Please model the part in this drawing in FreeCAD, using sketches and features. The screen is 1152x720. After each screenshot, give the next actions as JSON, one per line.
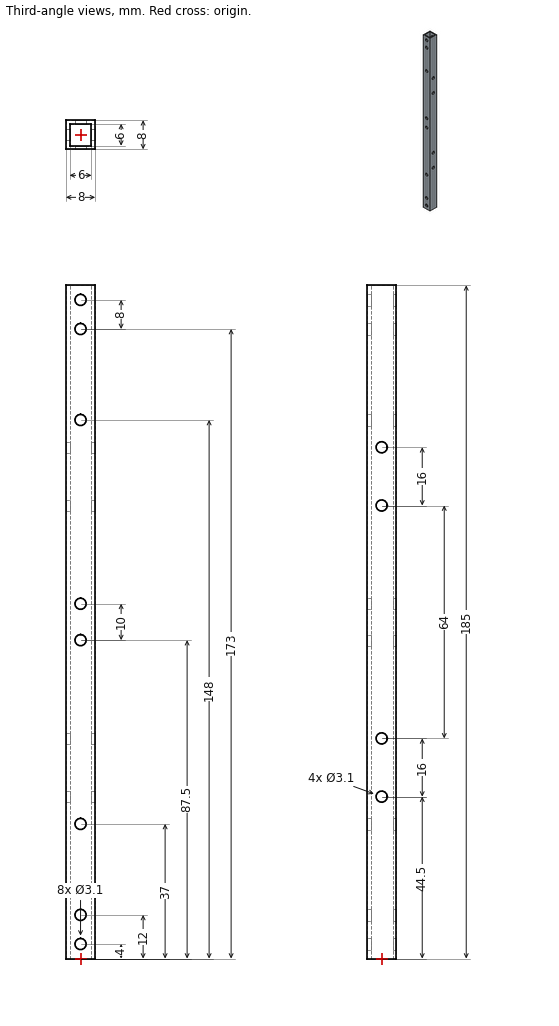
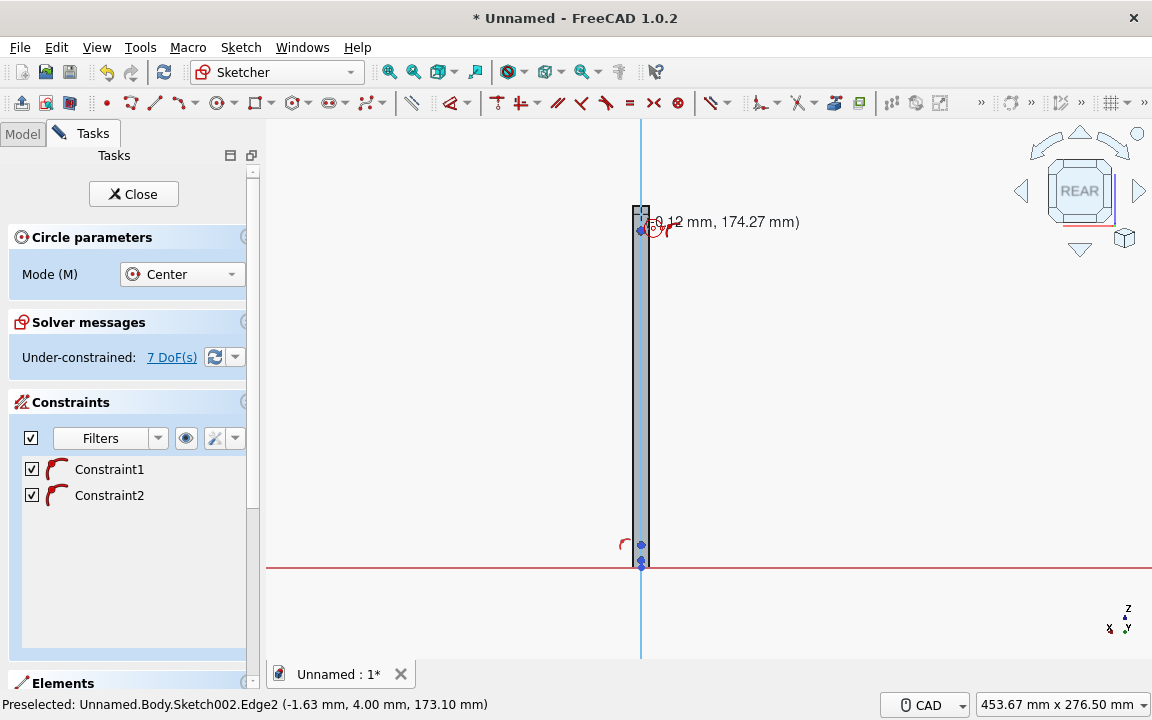
{"action": "scroll", "coordinate": [641, 214], "scroll_direction": "up", "scroll_amount": 2}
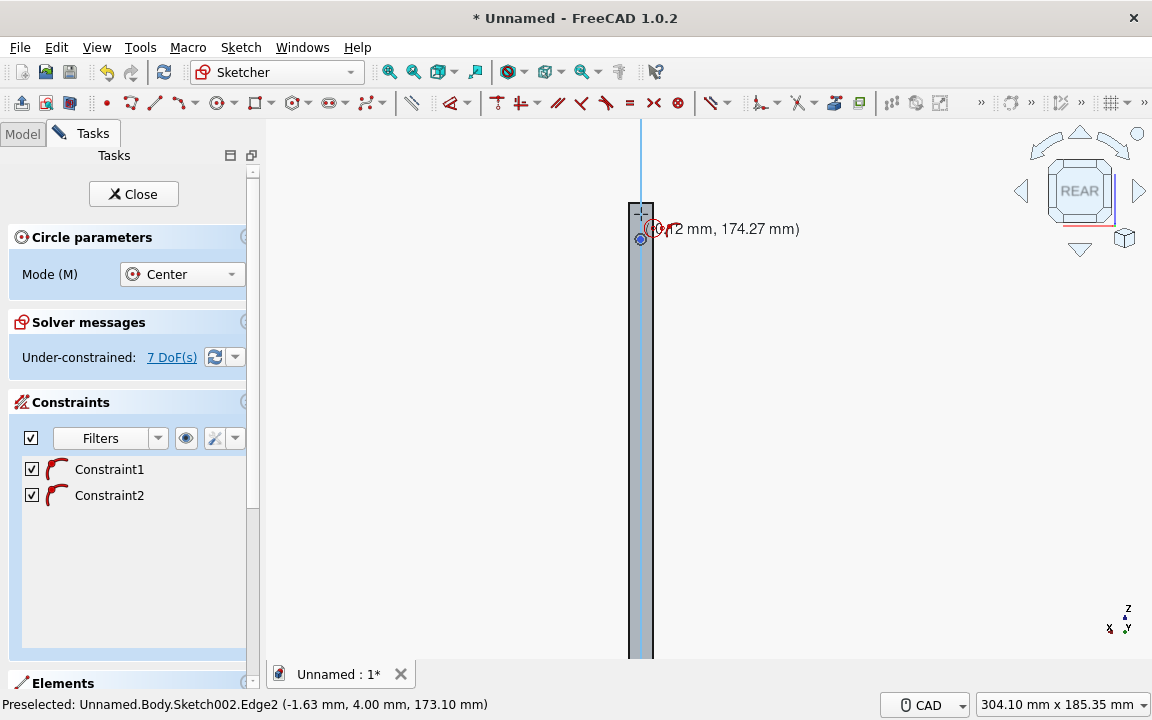
{"action": "left_click", "coordinate": [641, 214]}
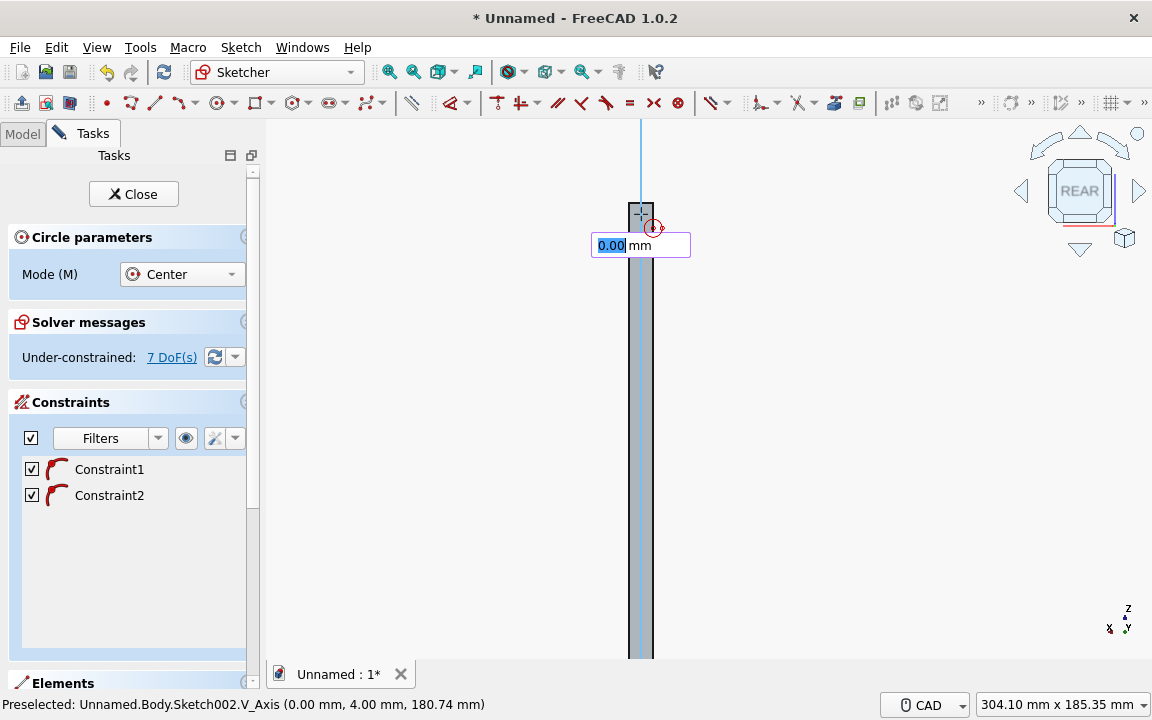
{"action": "scroll", "coordinate": [645, 213], "scroll_direction": "up", "scroll_amount": 7}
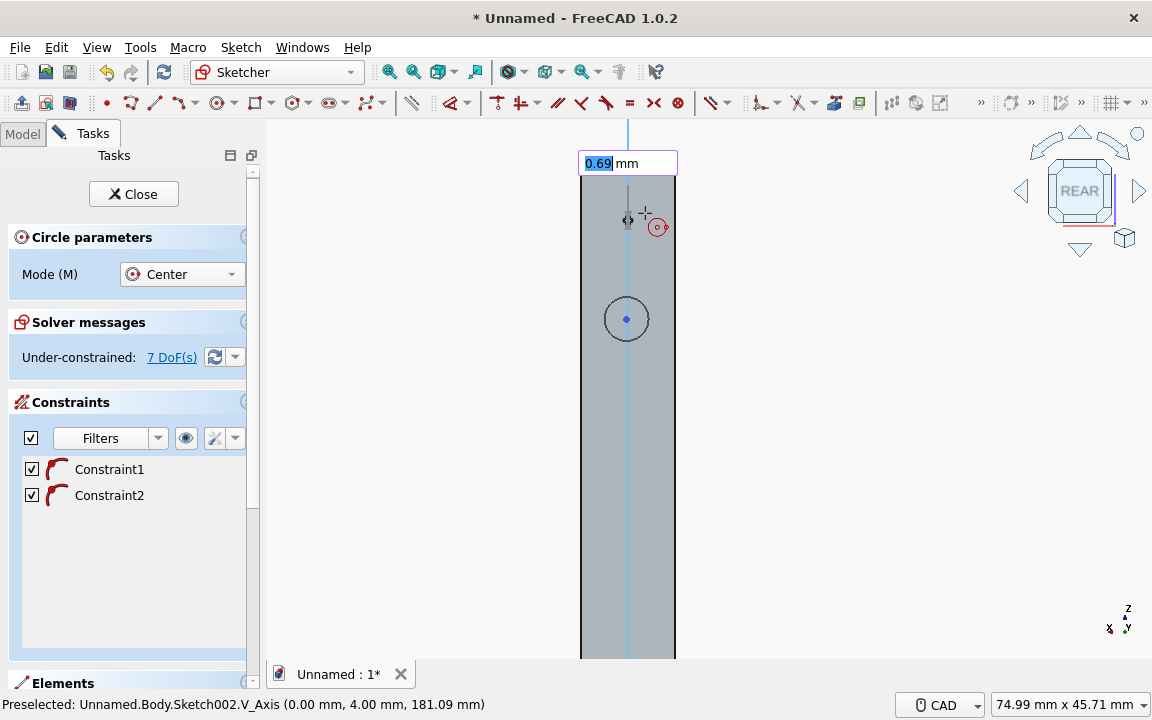
{"action": "left_click", "coordinate": [645, 211]}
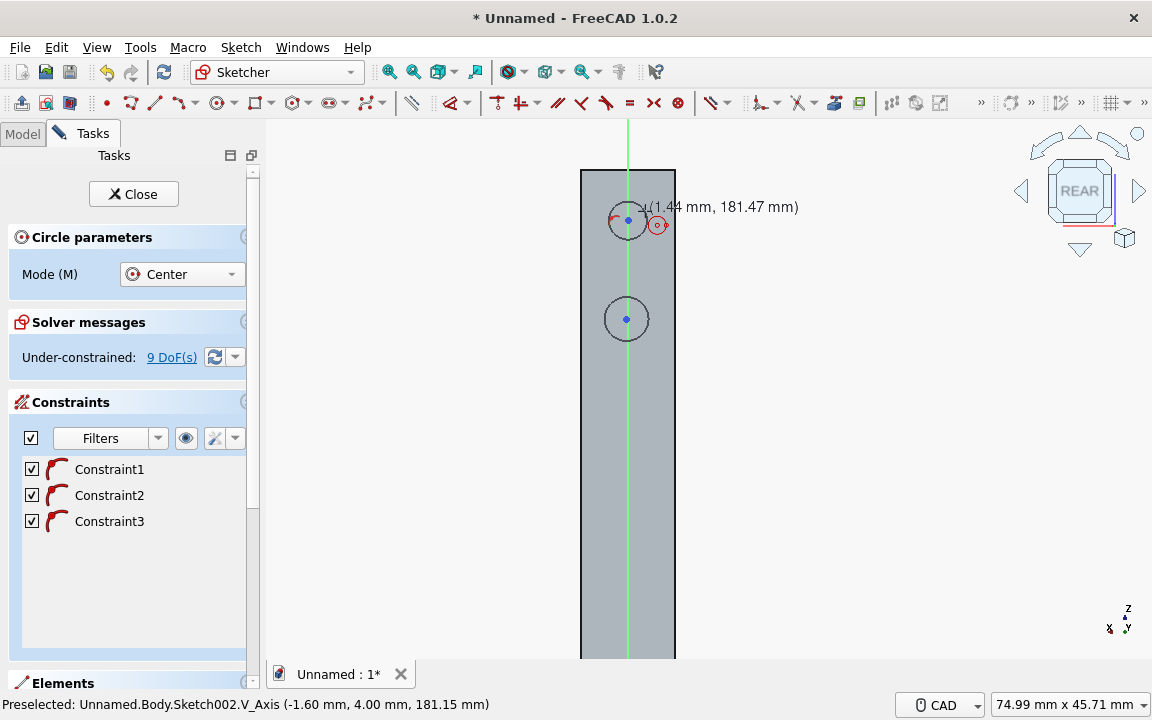
{"action": "scroll", "coordinate": [643, 213], "scroll_direction": "down", "scroll_amount": 9}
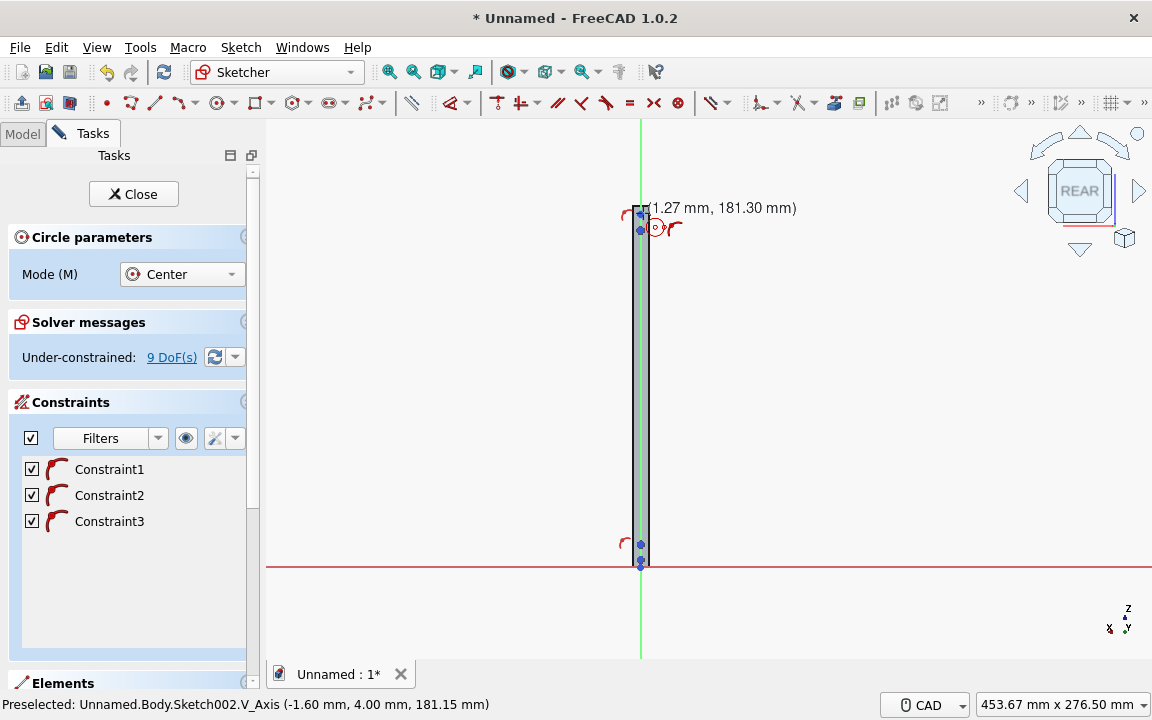
{"action": "scroll", "coordinate": [641, 396], "scroll_direction": "up", "scroll_amount": 11}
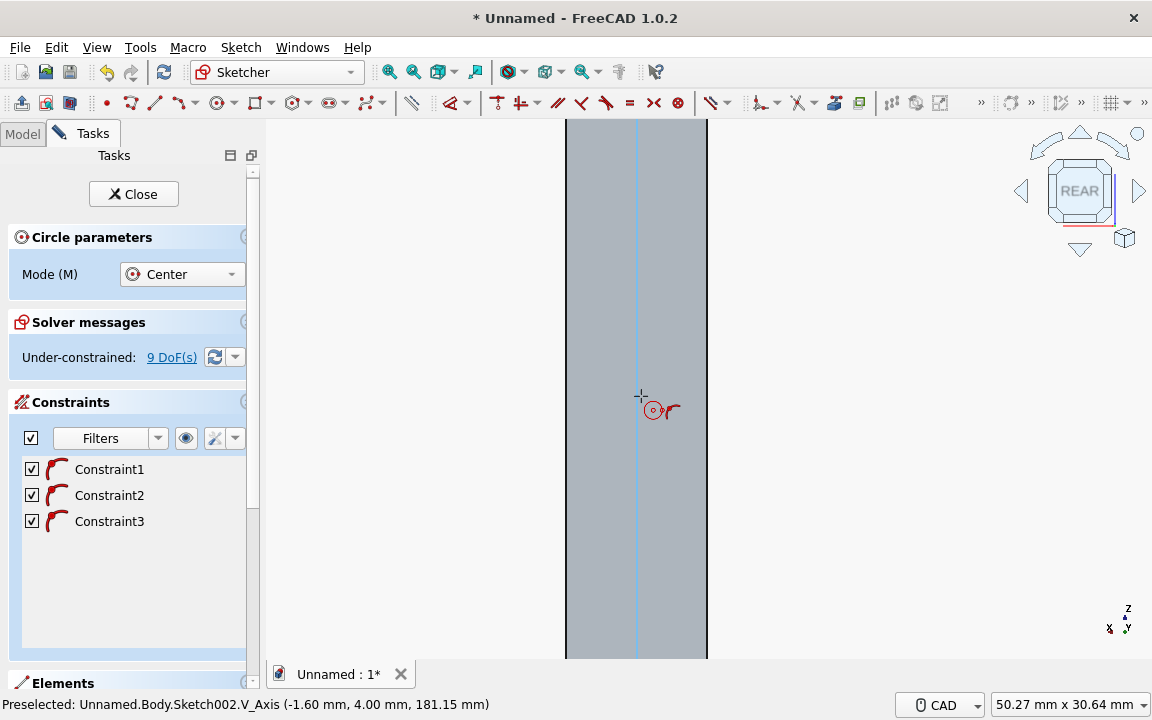
{"action": "scroll", "coordinate": [641, 396], "scroll_direction": "down", "scroll_amount": 11}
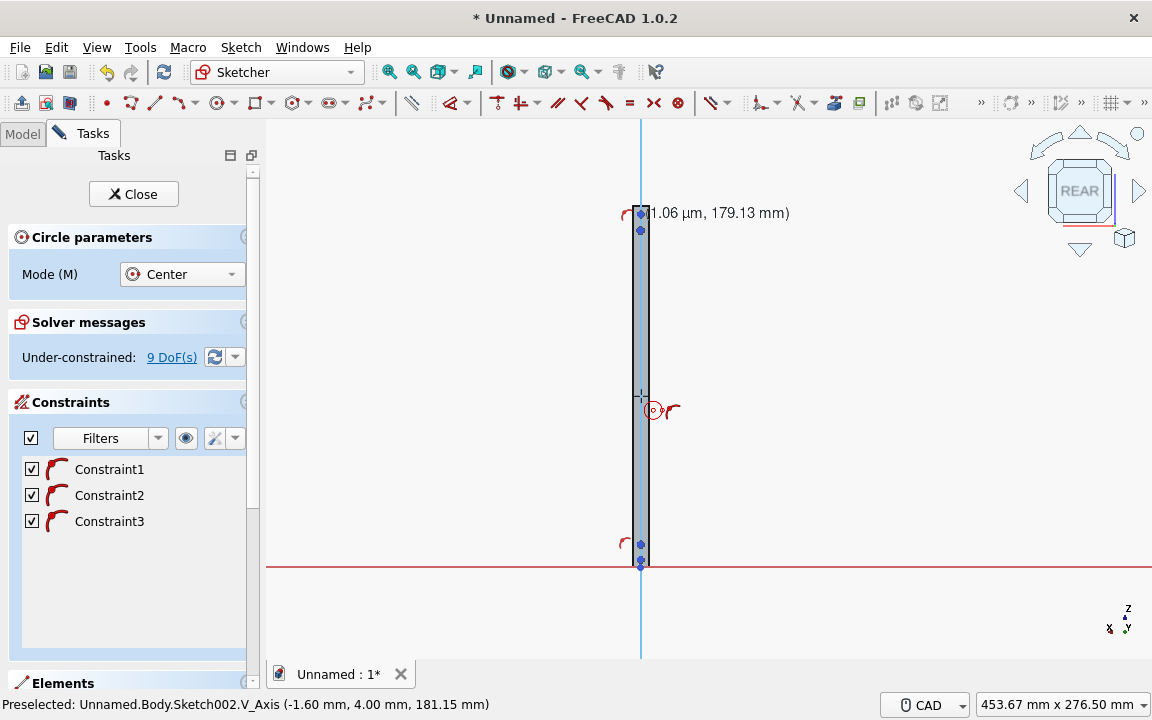
{"action": "left_click", "coordinate": [641, 396]}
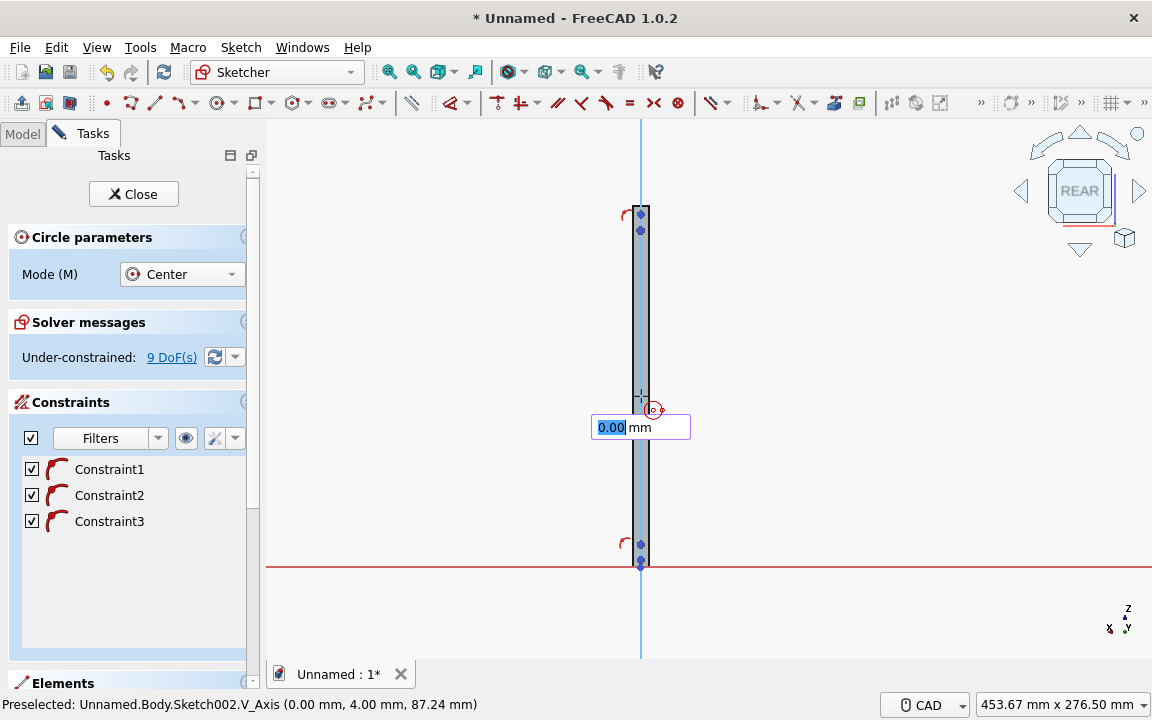
{"action": "scroll", "coordinate": [644, 395], "scroll_direction": "up", "scroll_amount": 9}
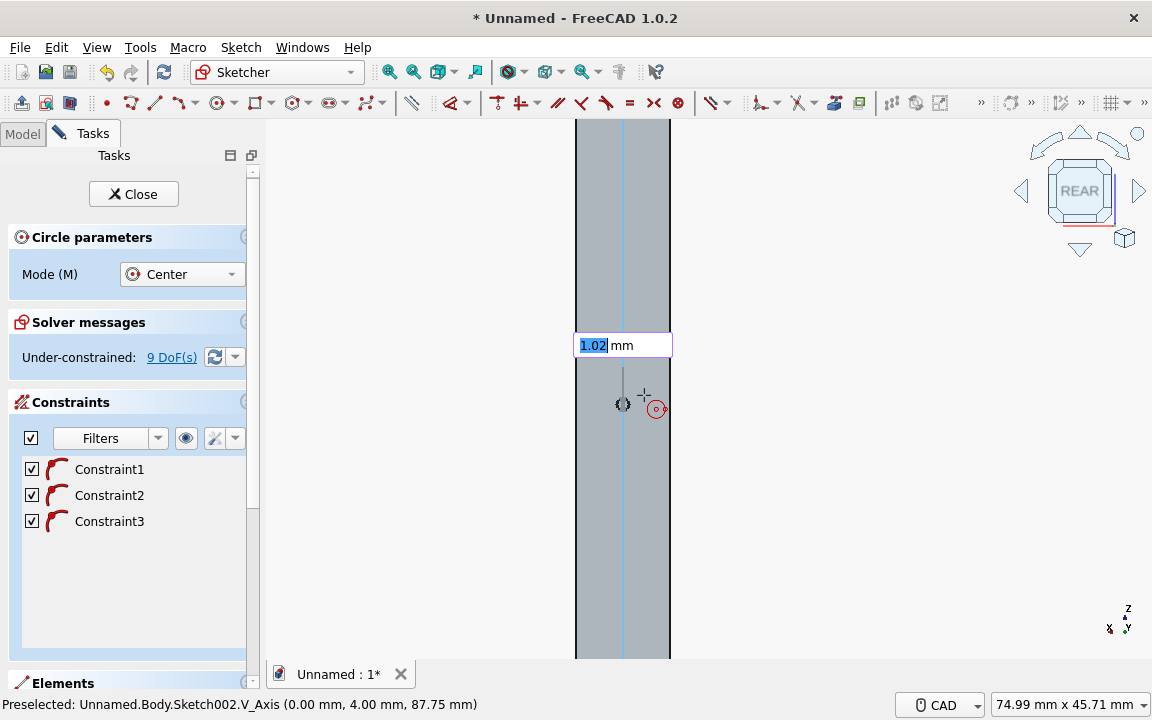
{"action": "left_click", "coordinate": [640, 395]}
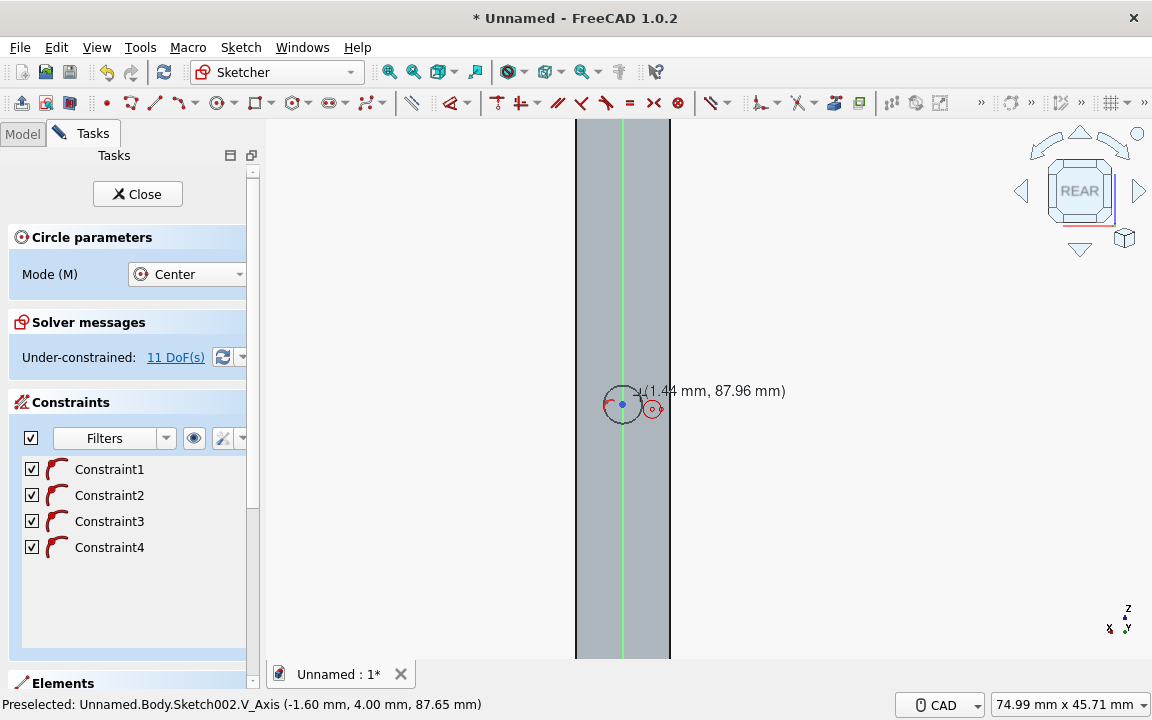
{"action": "scroll", "coordinate": [623, 283], "scroll_direction": "up", "scroll_amount": 2}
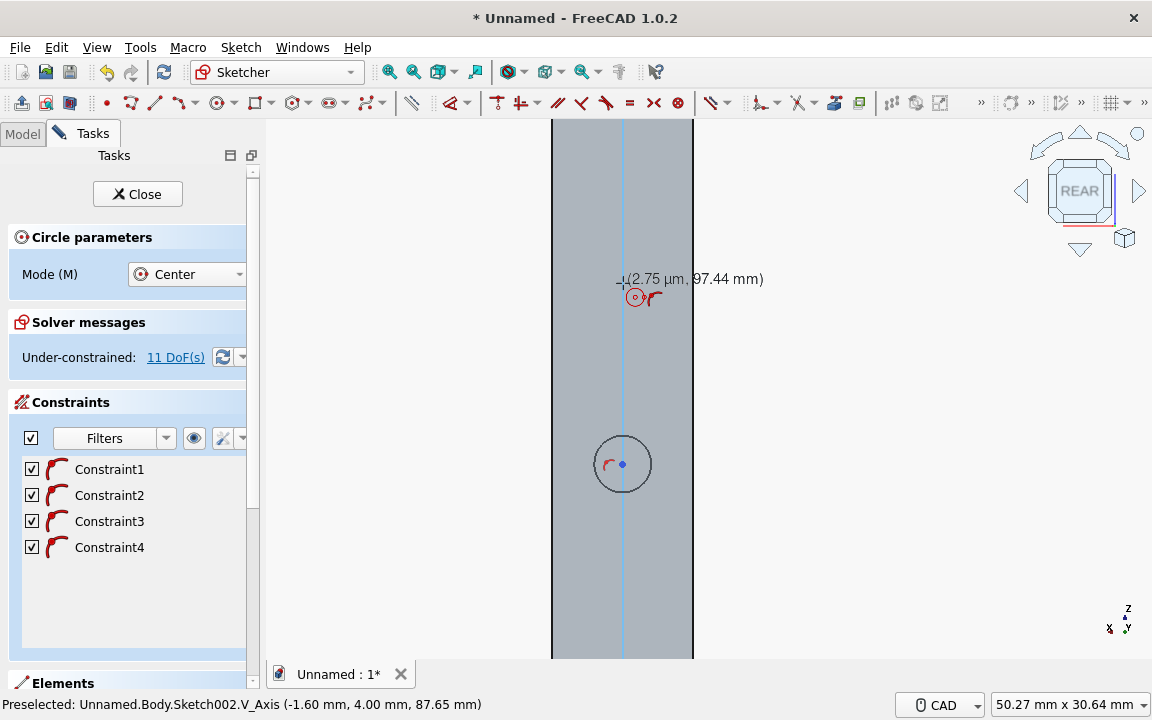
{"action": "scroll", "coordinate": [643, 388], "scroll_direction": "down", "scroll_amount": 11}